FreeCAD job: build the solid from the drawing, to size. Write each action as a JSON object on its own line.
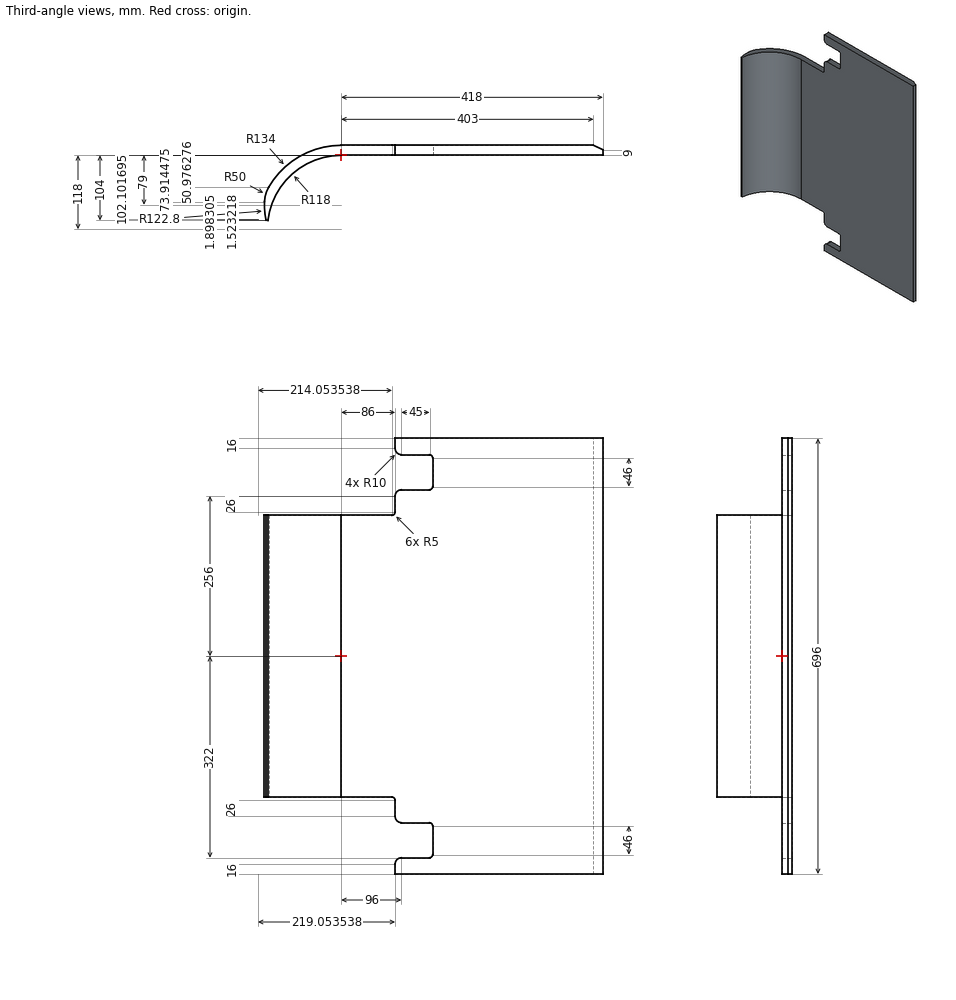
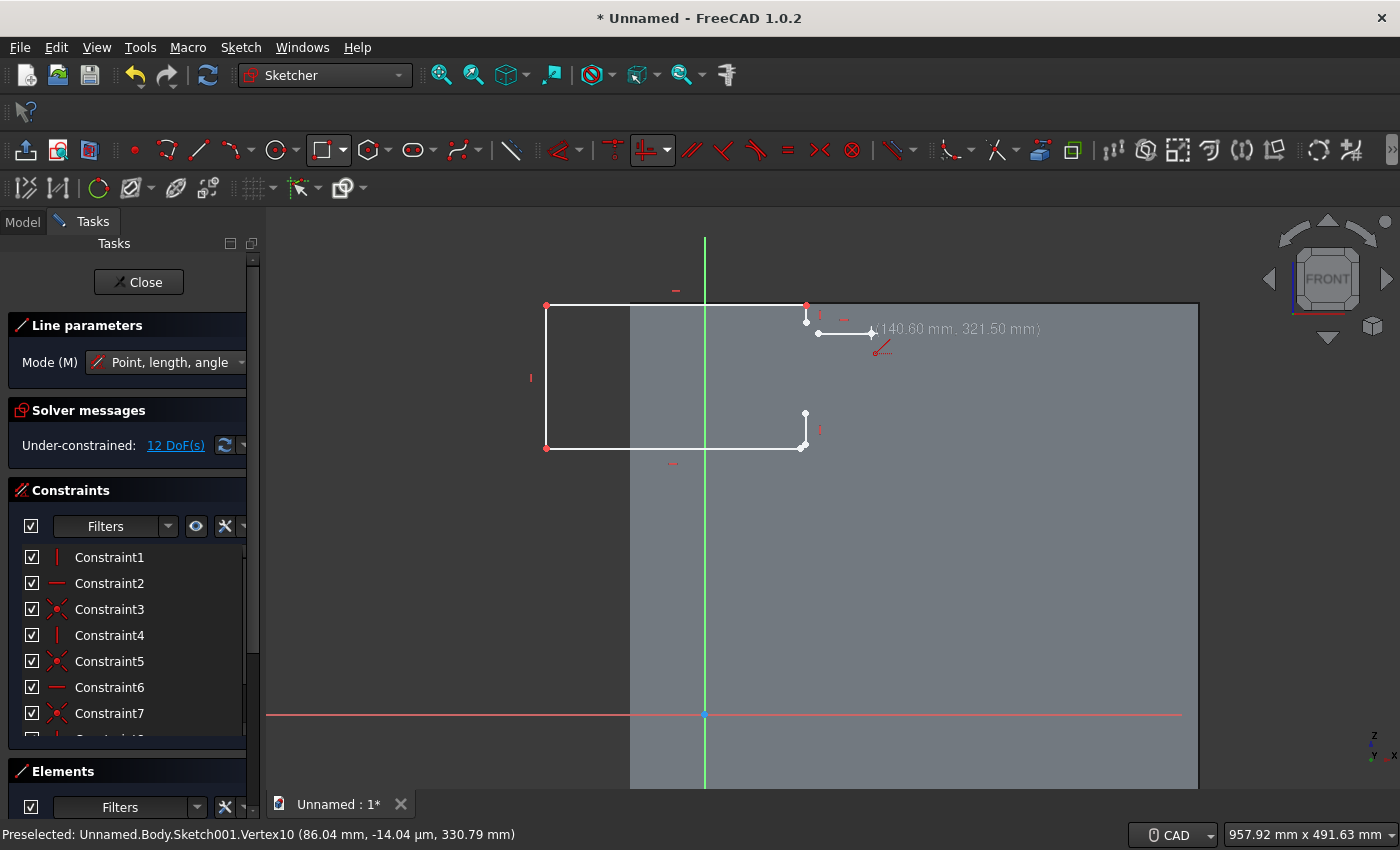
{"action": "scroll", "coordinate": [877, 339], "scroll_direction": "up", "scroll_amount": 4}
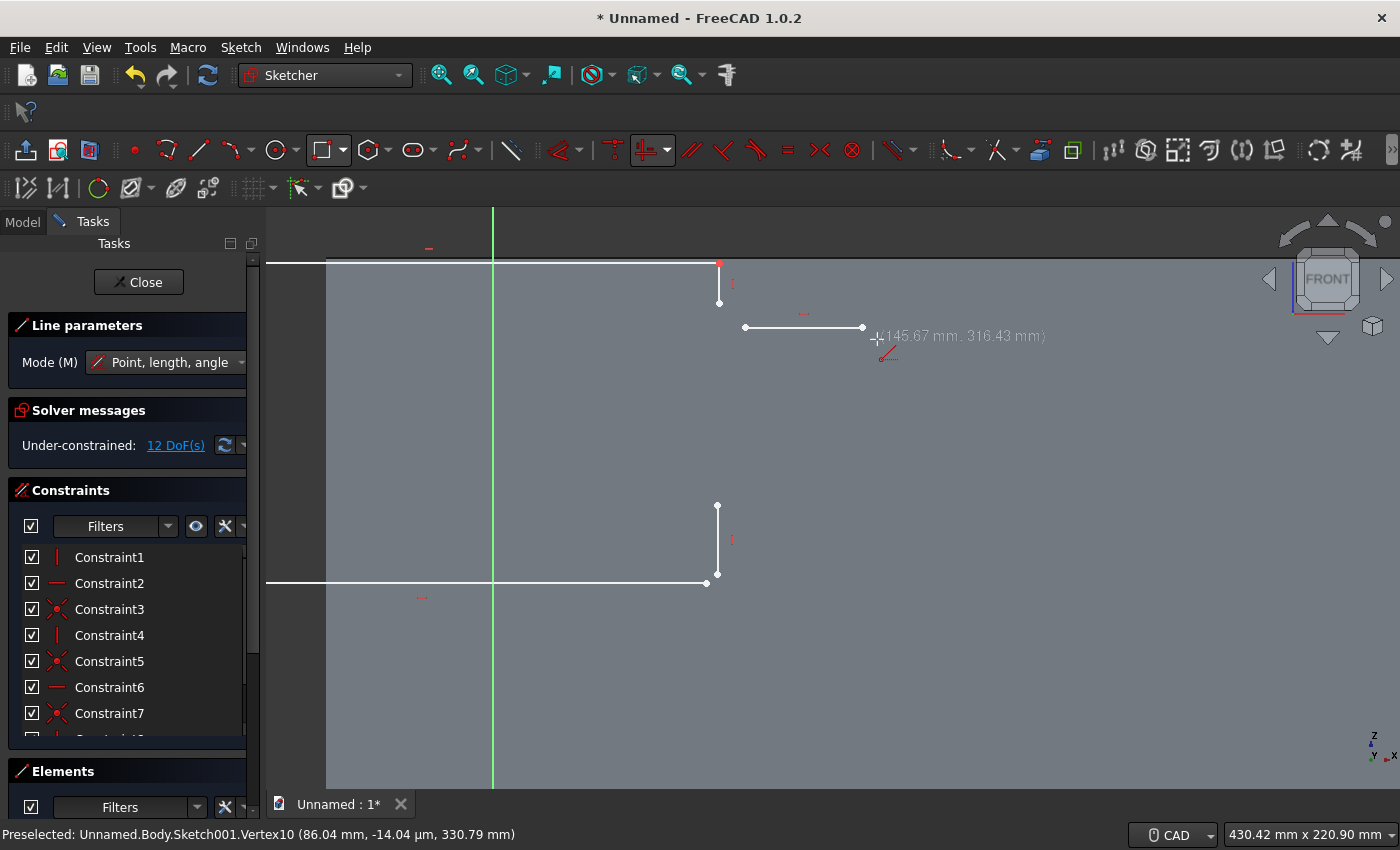
{"action": "left_click", "coordinate": [877, 339]}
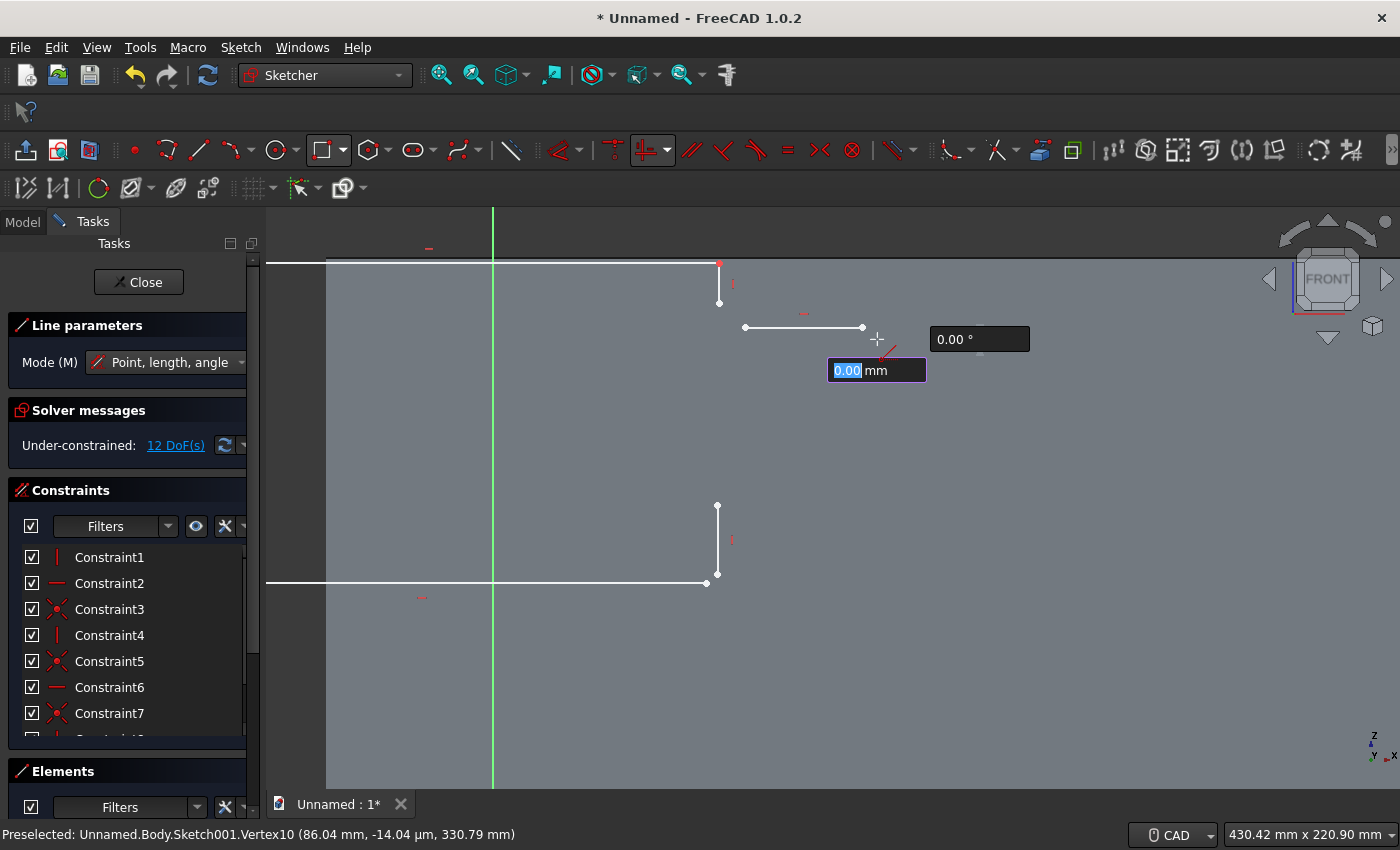
{"action": "scroll", "coordinate": [829, 327], "scroll_direction": "down", "scroll_amount": 8}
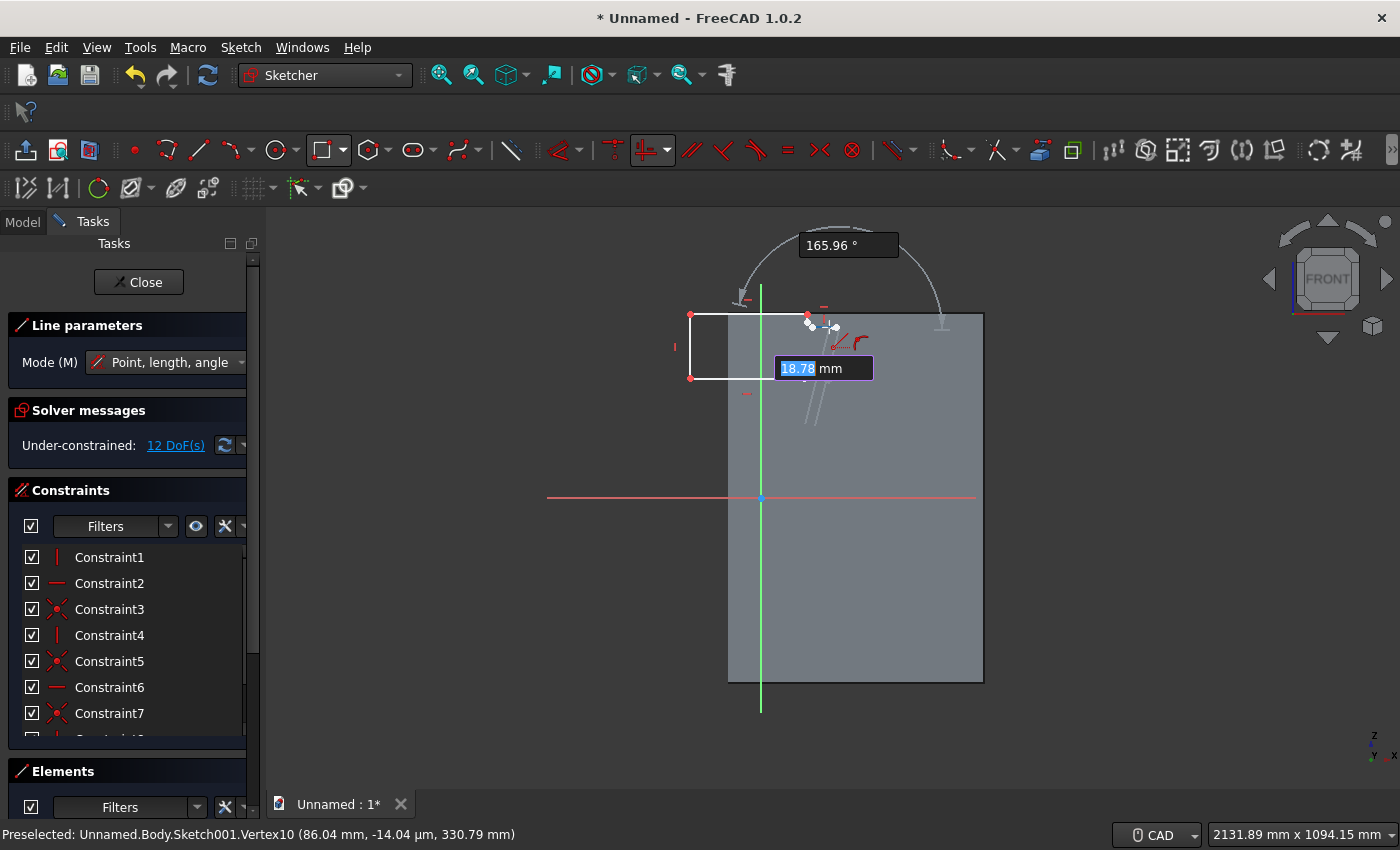
{"action": "left_click", "coordinate": [839, 354]}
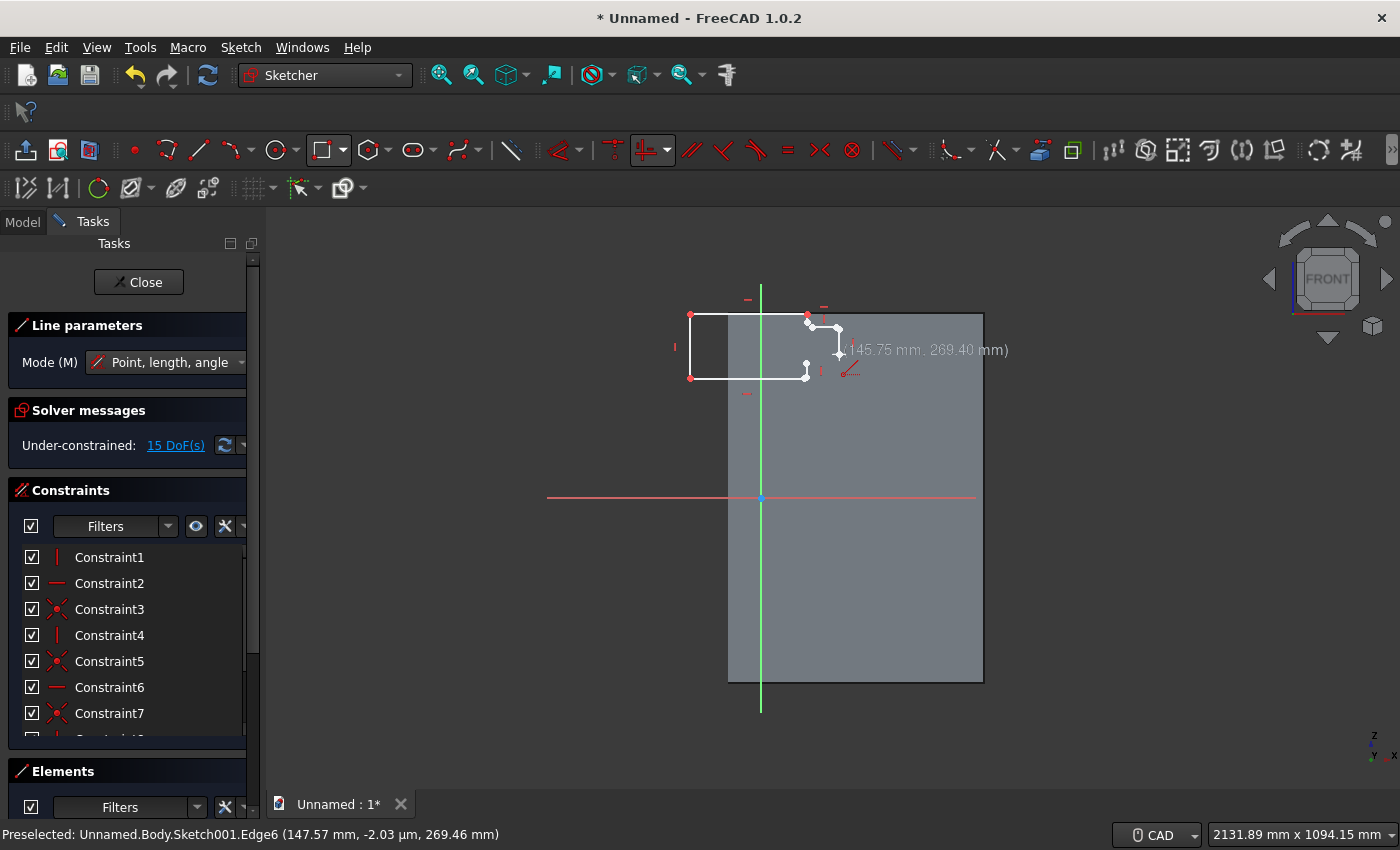
{"action": "scroll", "coordinate": [836, 357], "scroll_direction": "up", "scroll_amount": 8}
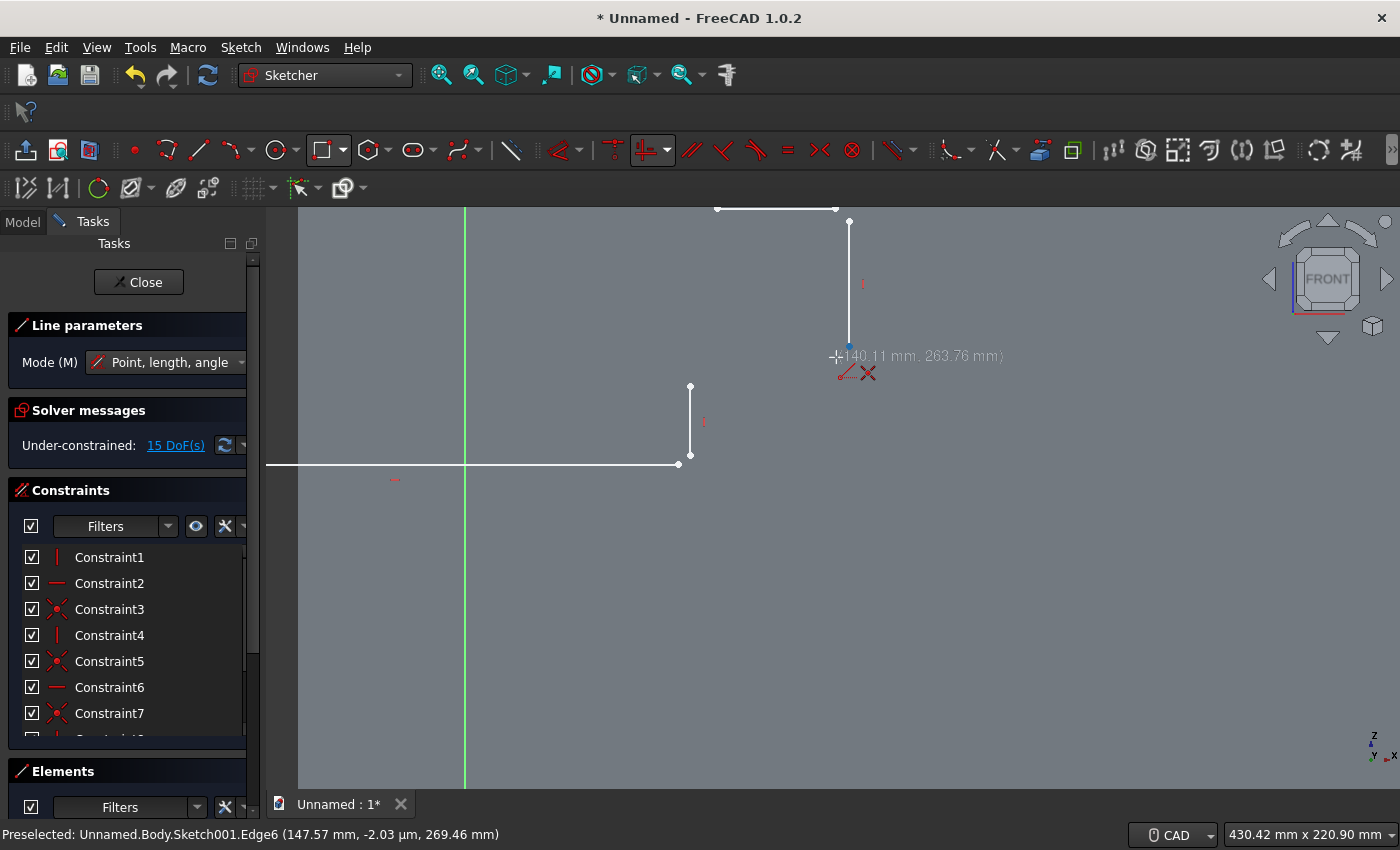
{"action": "left_click", "coordinate": [836, 355]}
{"action": "left_click", "coordinate": [718, 355]}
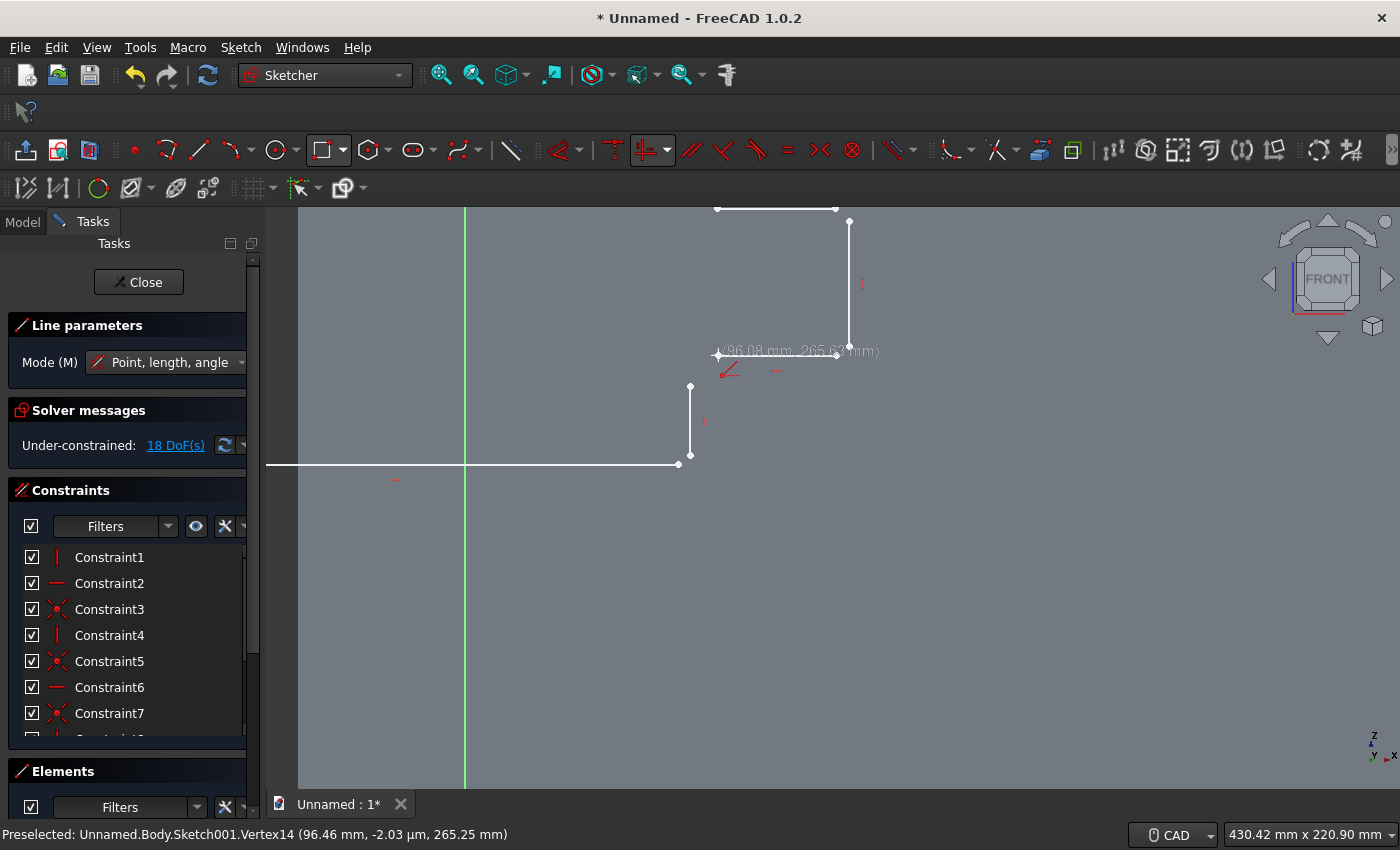
{"action": "left_click", "coordinate": [232, 150]}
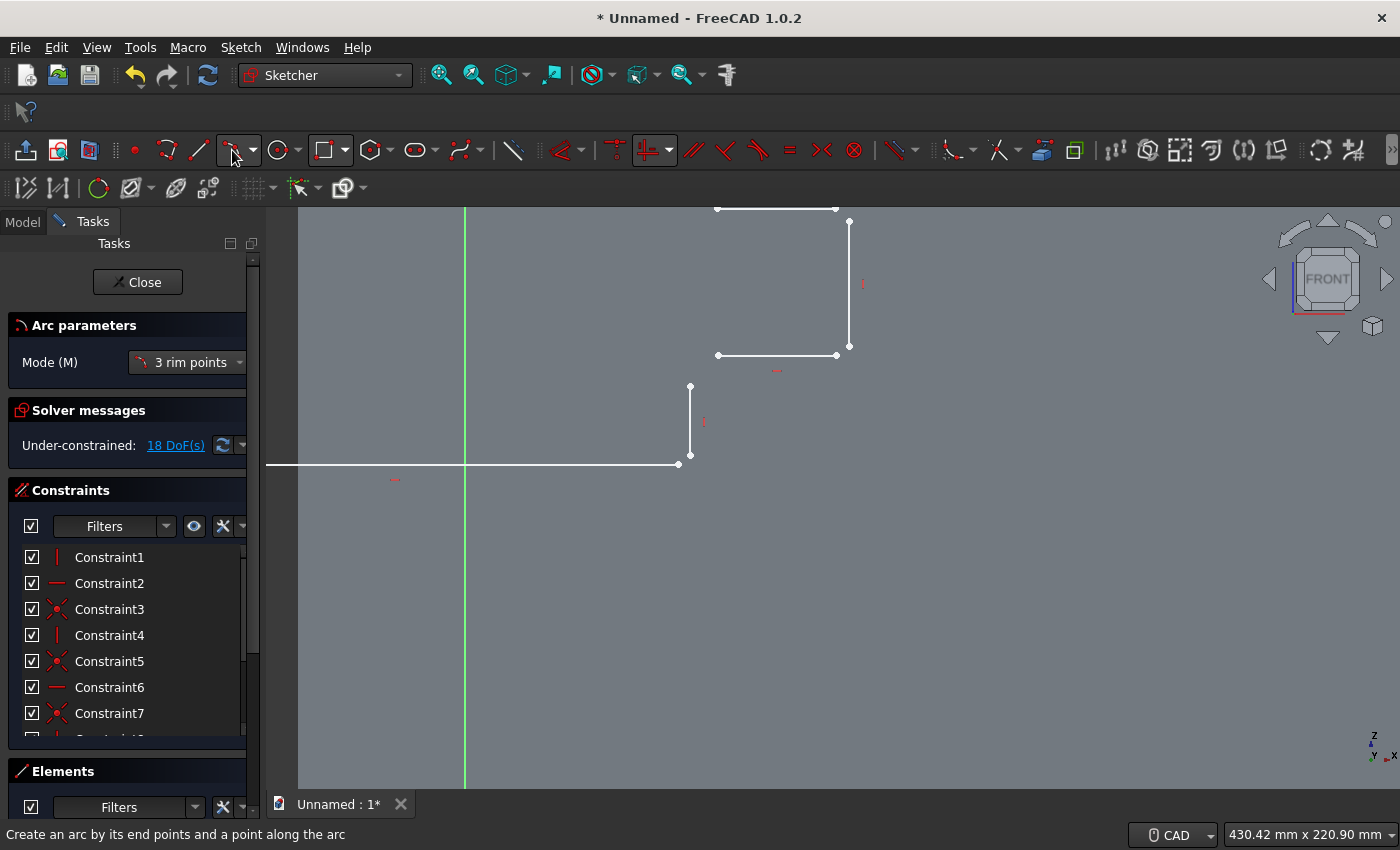
{"action": "left_click", "coordinate": [690, 456]}
{"action": "left_click", "coordinate": [678, 465]}